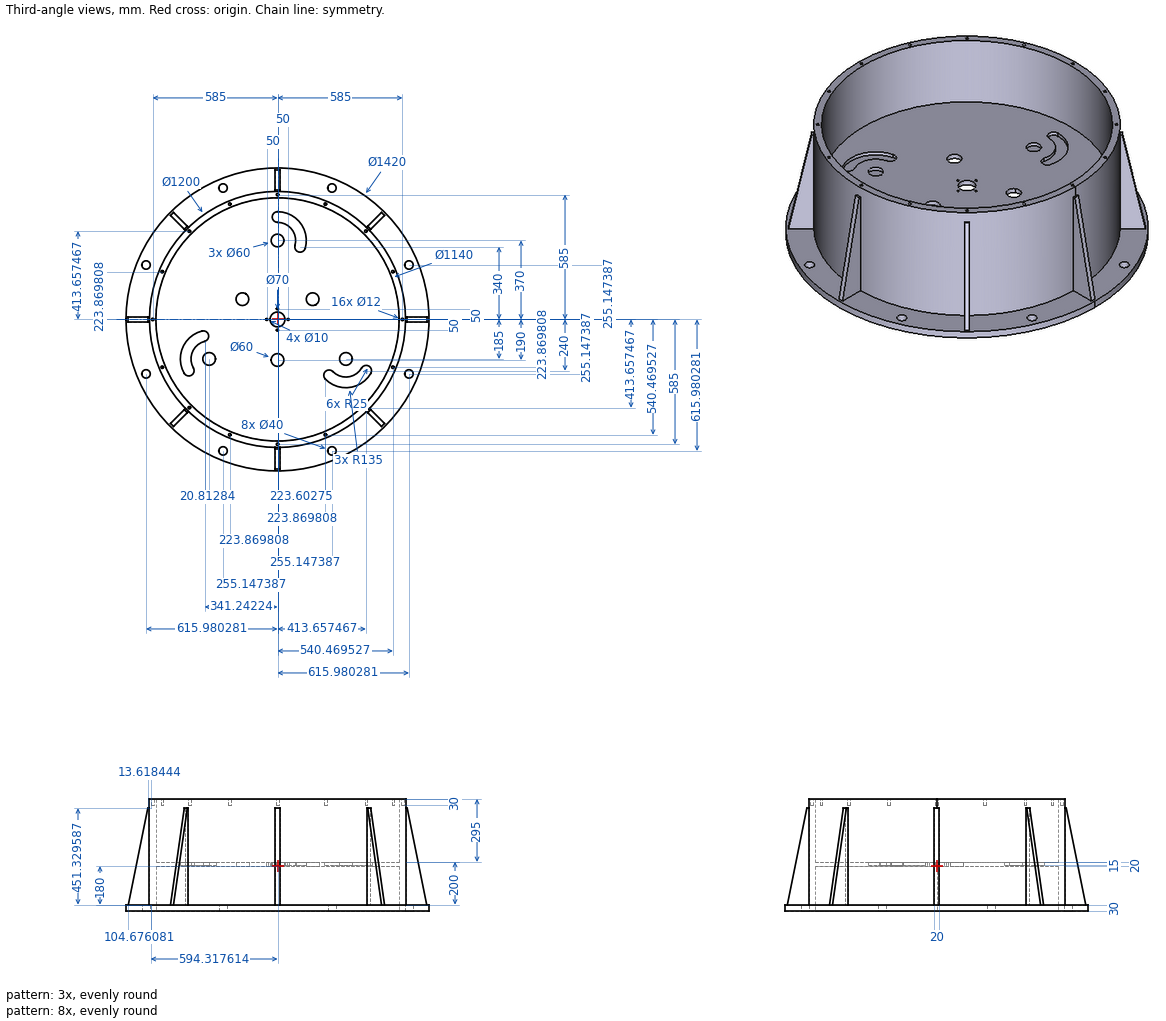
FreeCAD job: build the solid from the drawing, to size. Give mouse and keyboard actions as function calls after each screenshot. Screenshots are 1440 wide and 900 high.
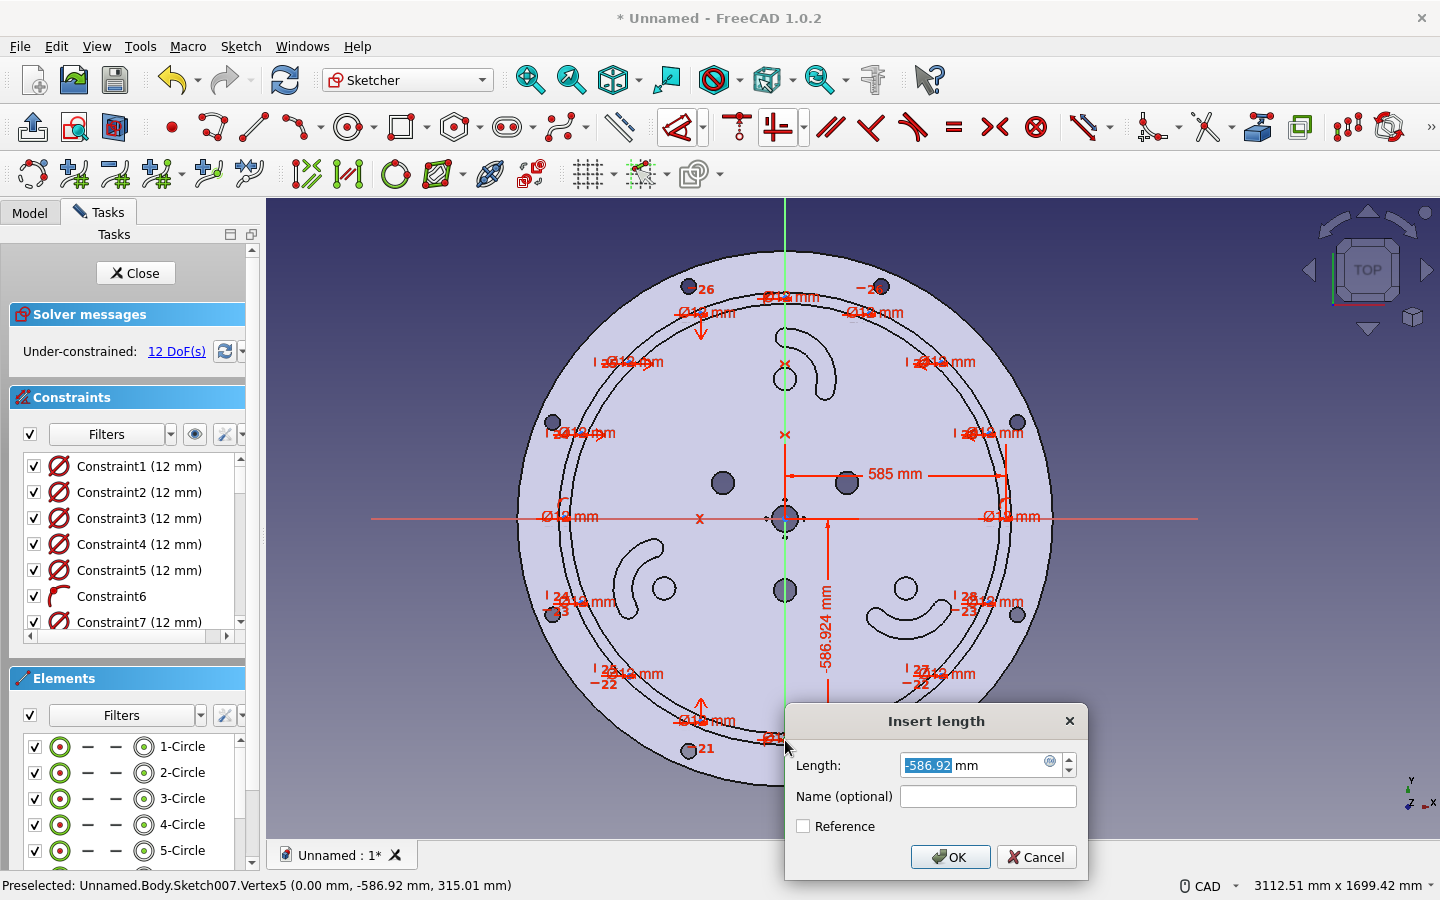
text(-585)
key(Return)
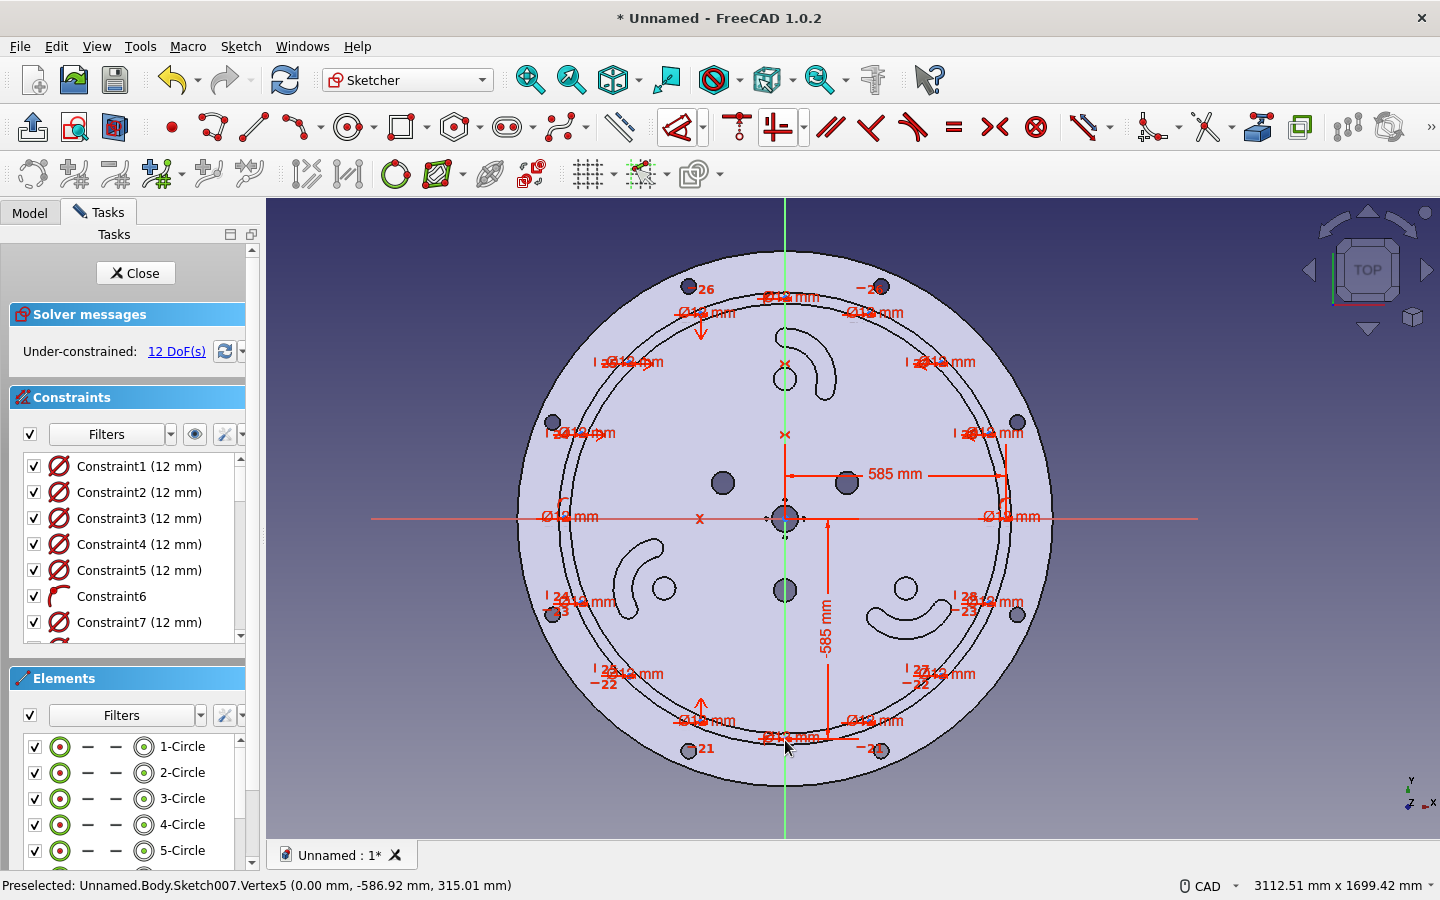
click(564, 519)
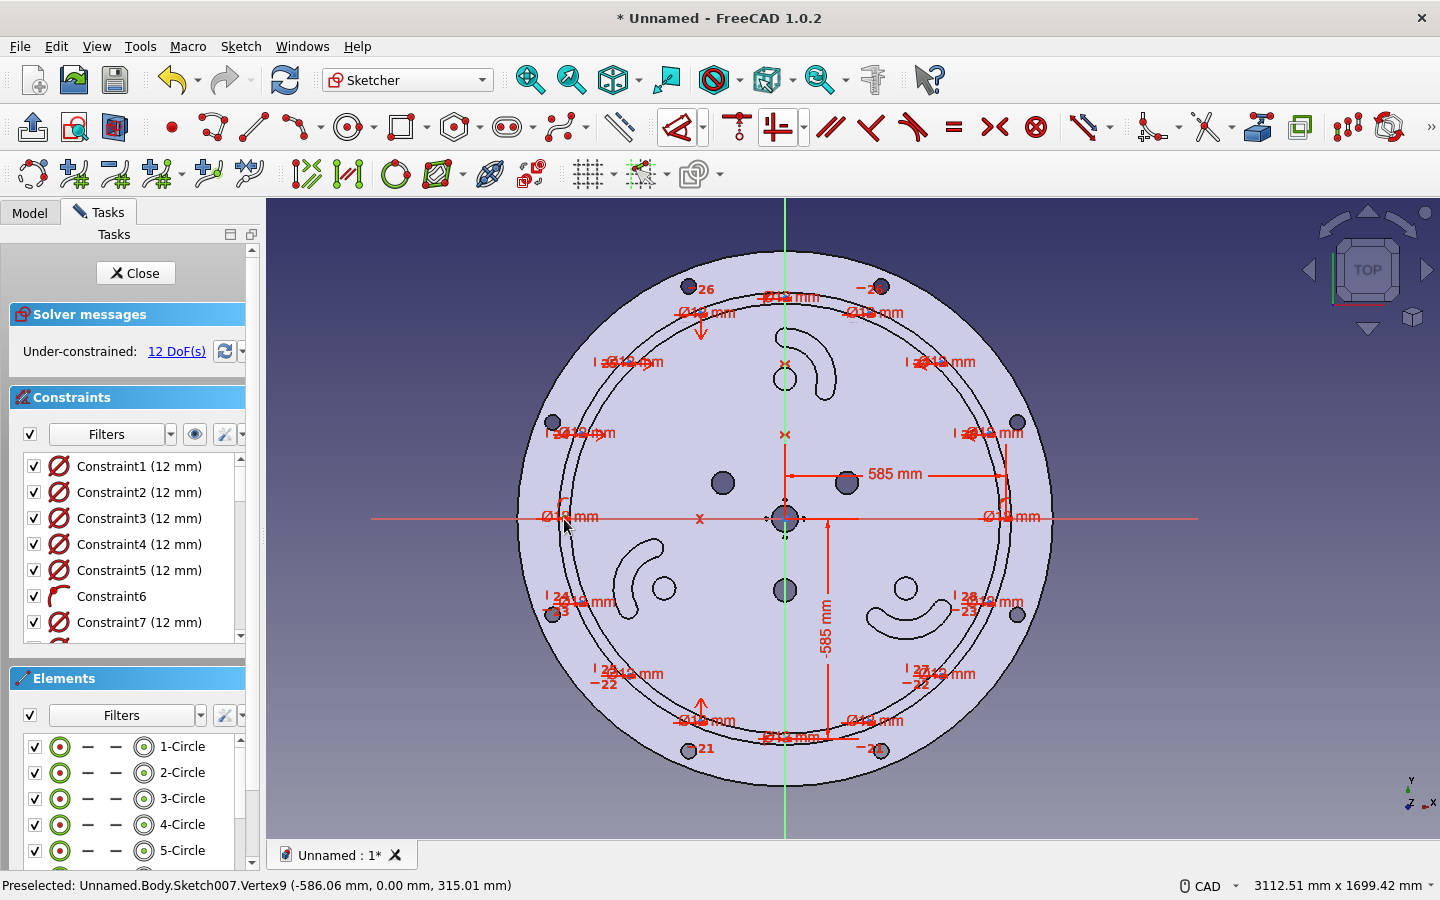
key(l)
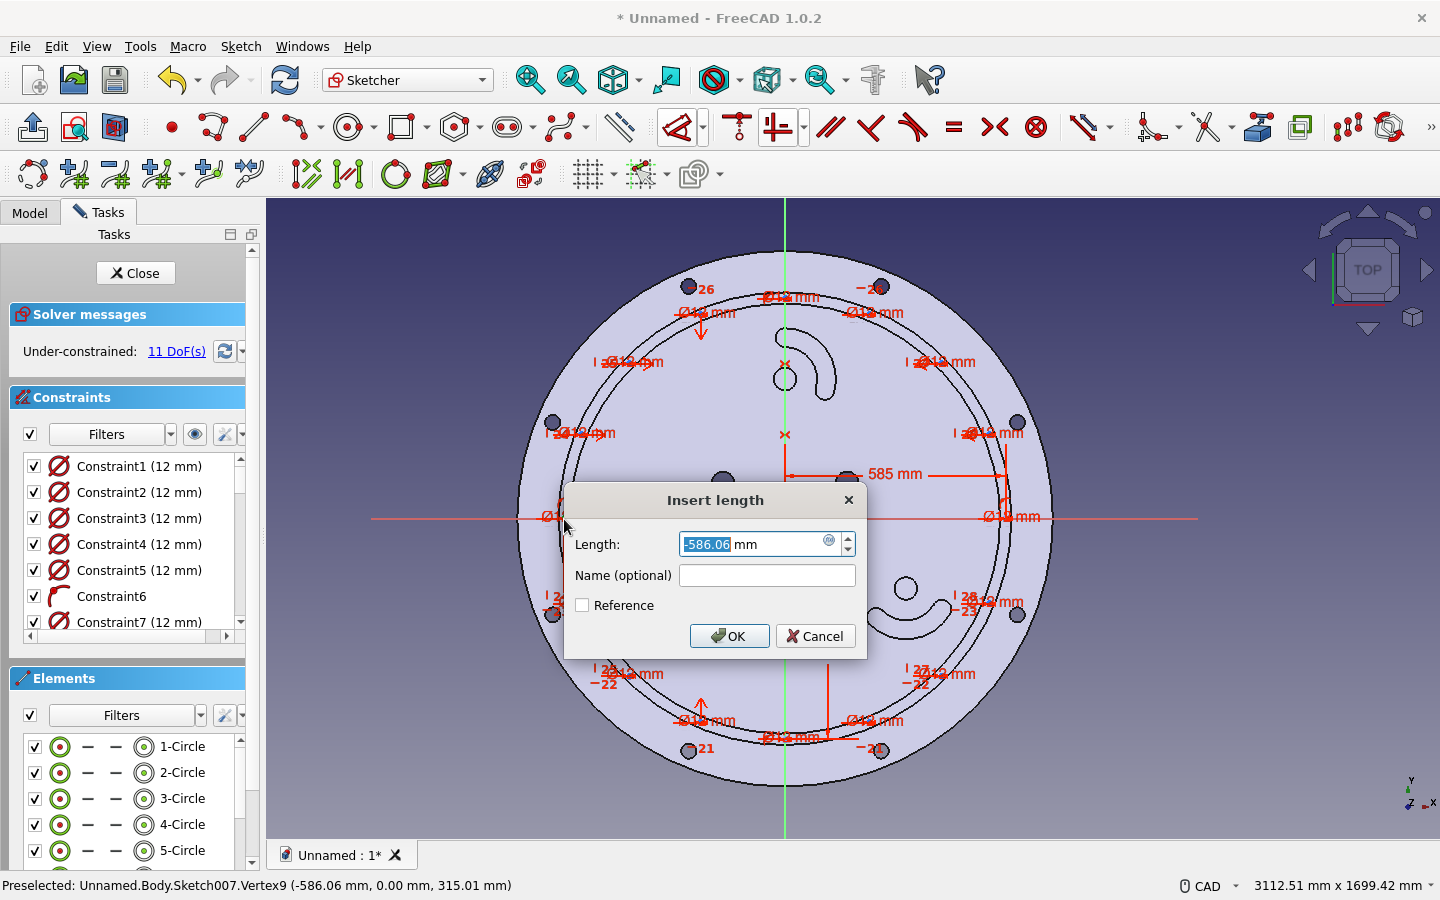
text(-585)
key(Return)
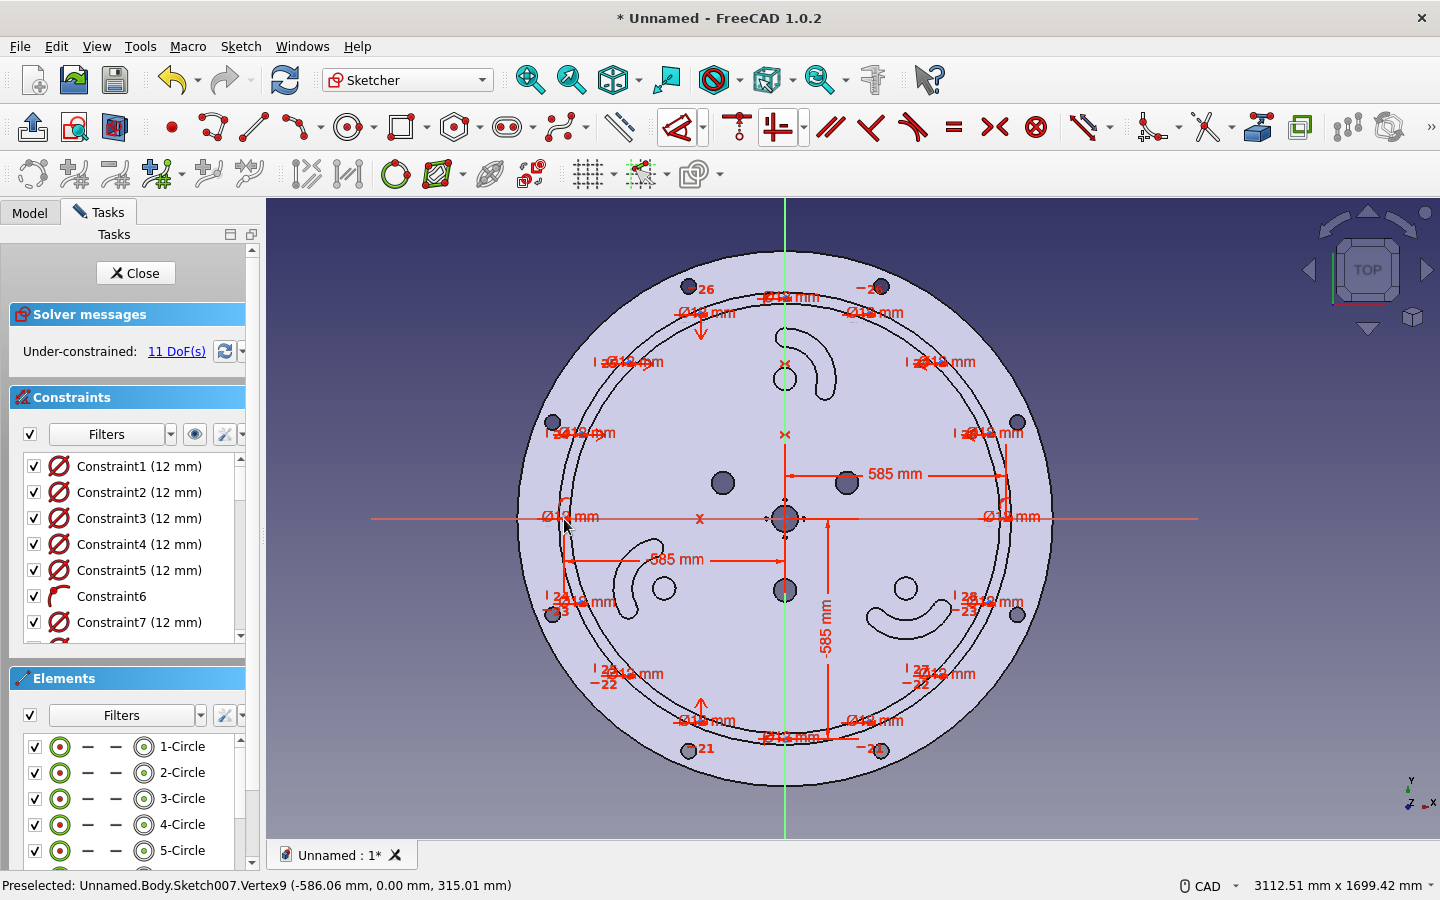
click(785, 299)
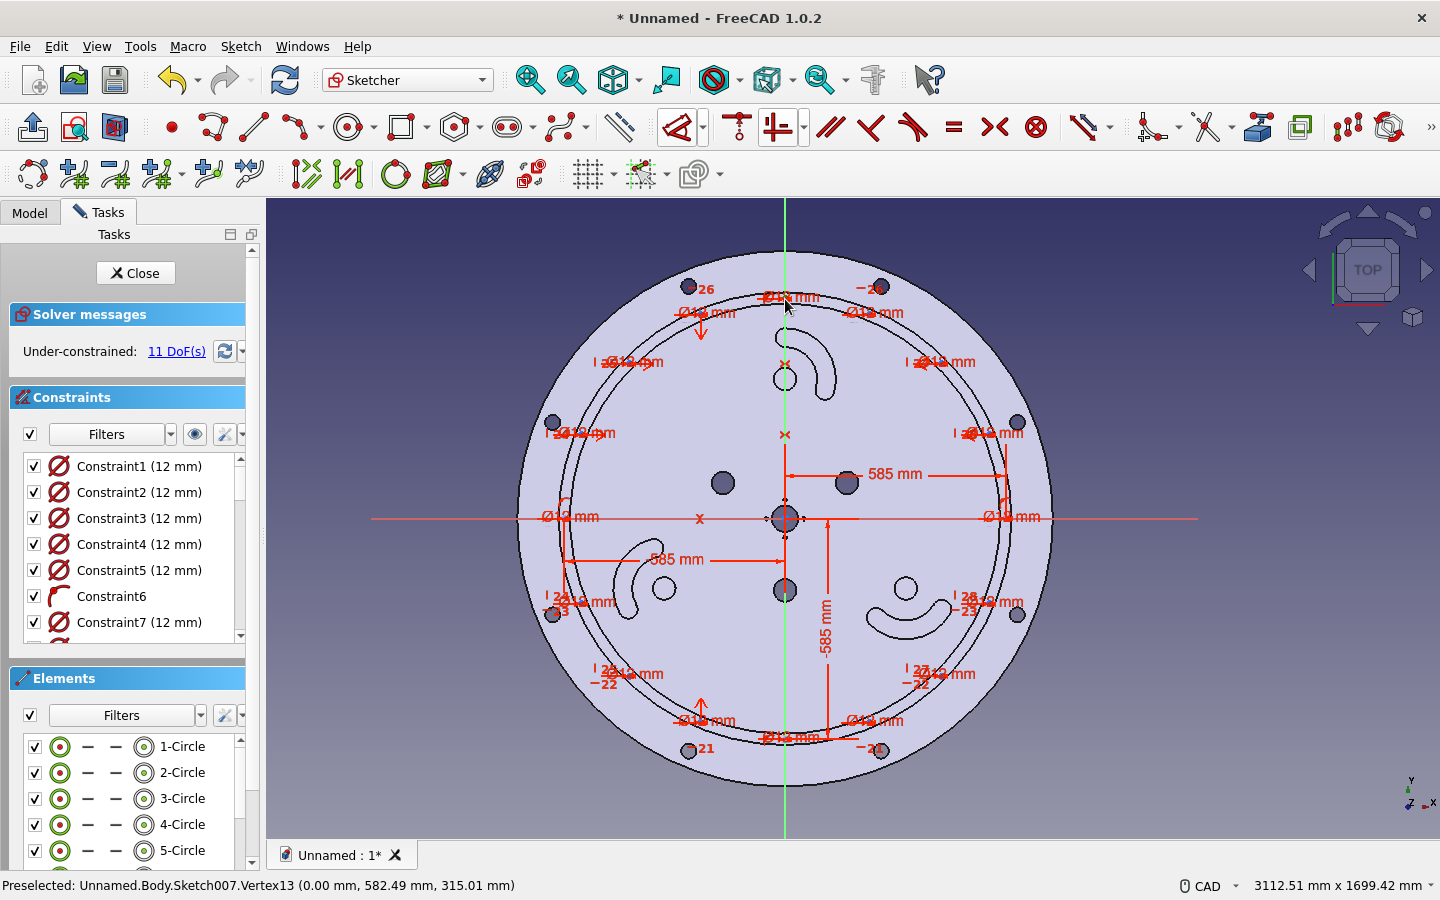
key(i)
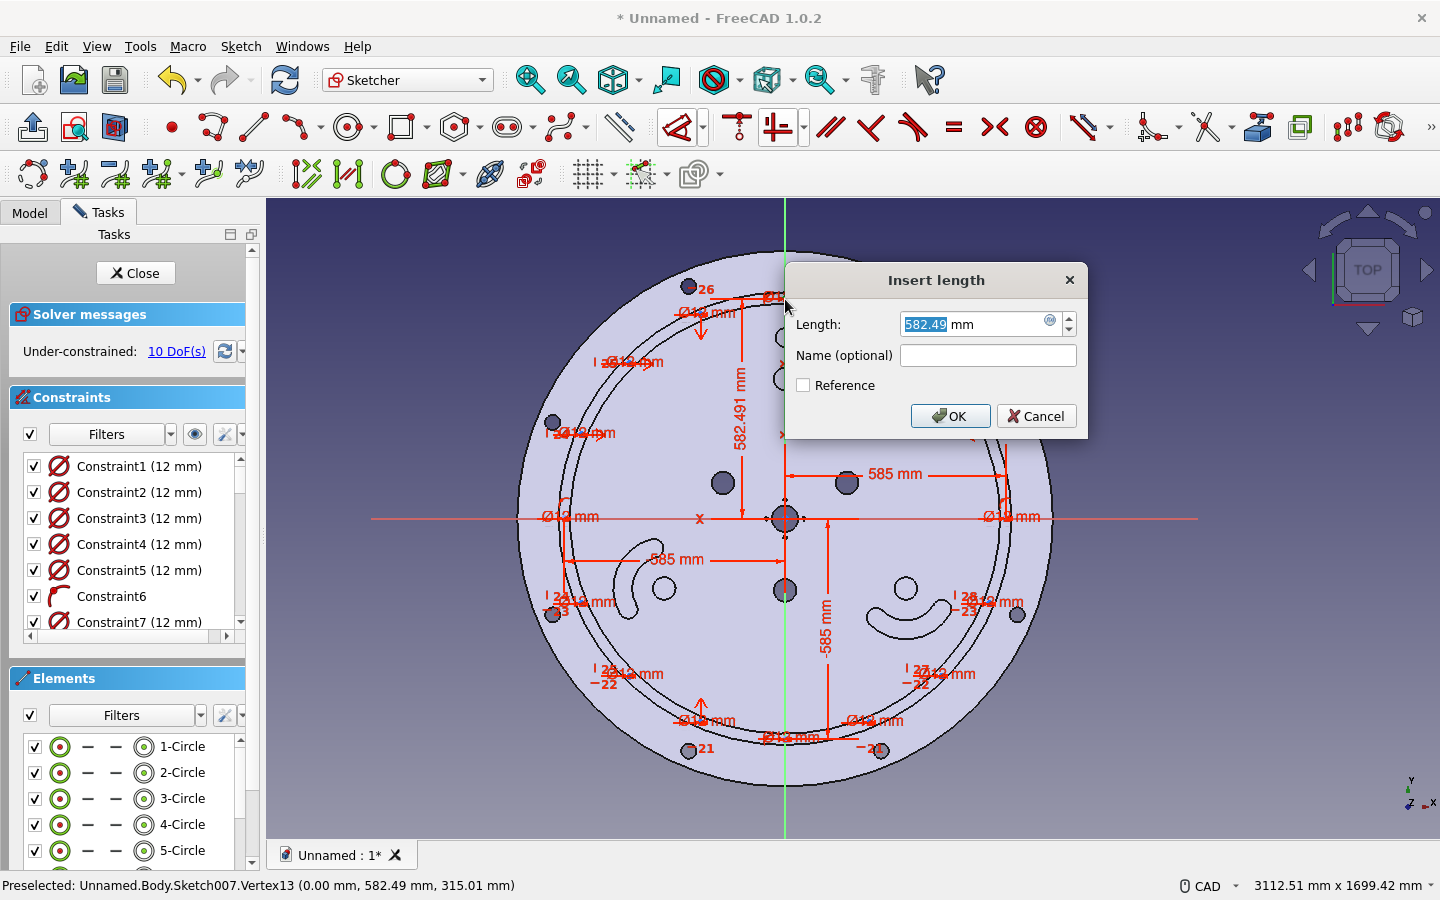
text(585)
key(Return)